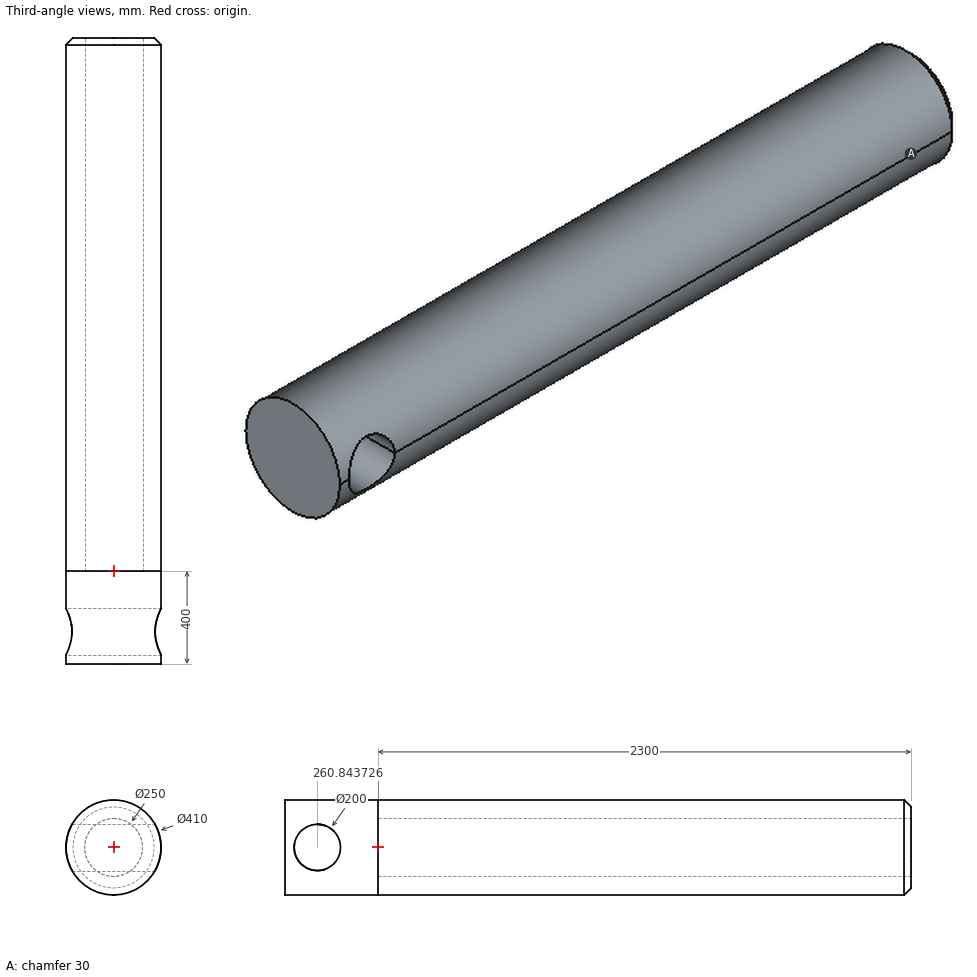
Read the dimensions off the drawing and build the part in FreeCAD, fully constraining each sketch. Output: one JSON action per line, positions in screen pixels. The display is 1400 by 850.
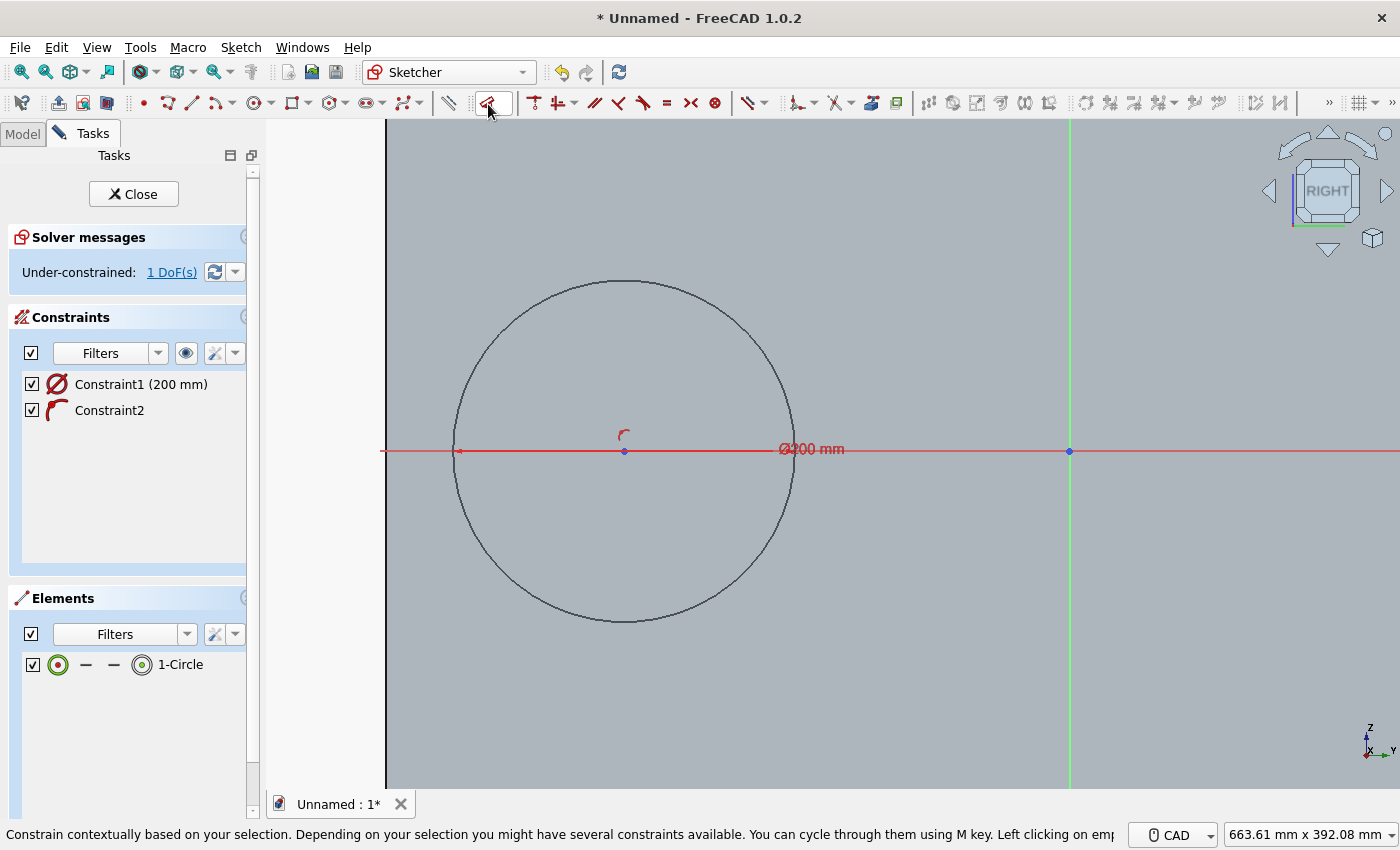
{"action": "left_click", "coordinate": [624, 451]}
{"action": "left_click", "coordinate": [847, 485]}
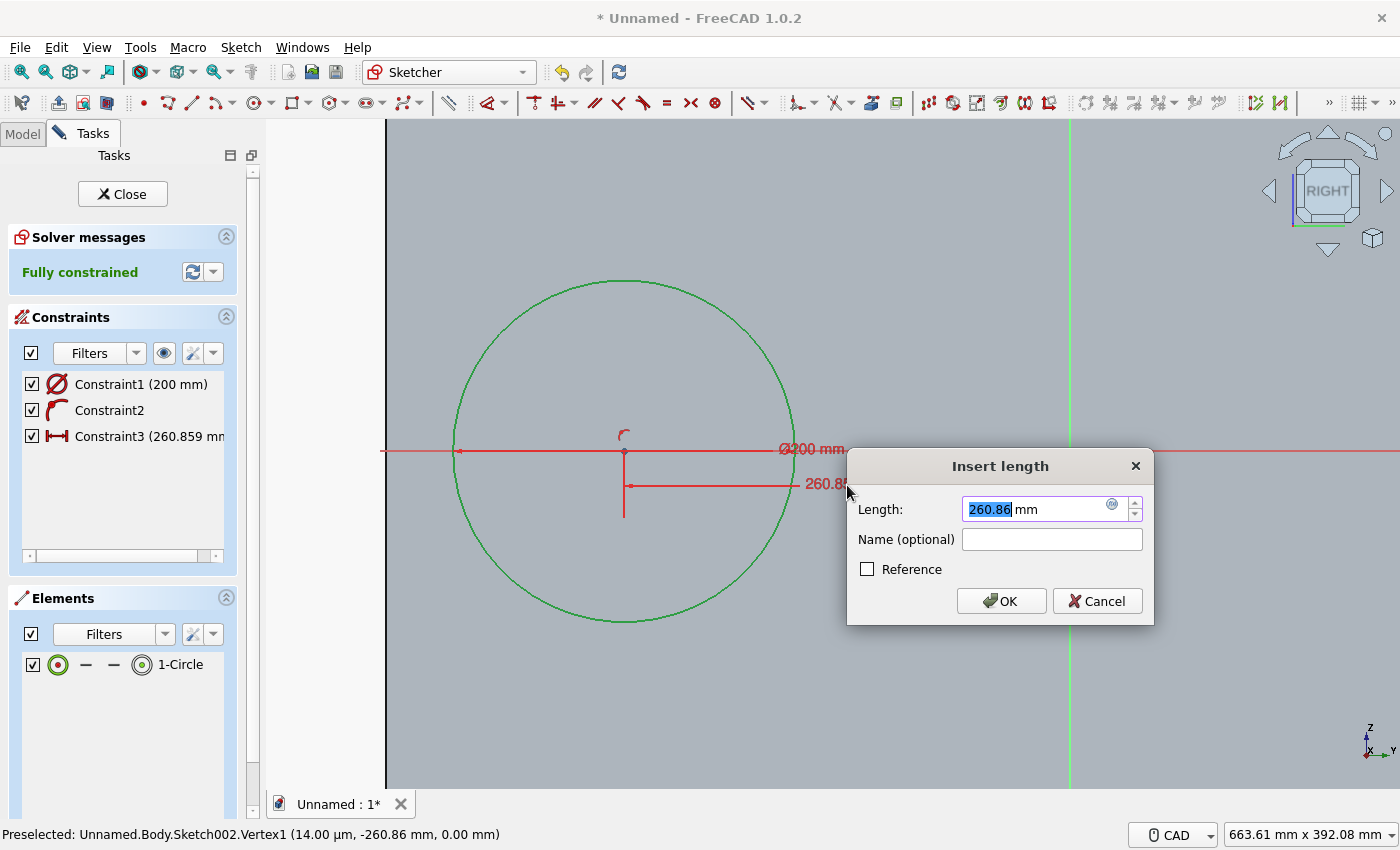
{"action": "type", "text": "260.843726"}
{"action": "key", "text": "Return"}
{"action": "key", "text": "Escape"}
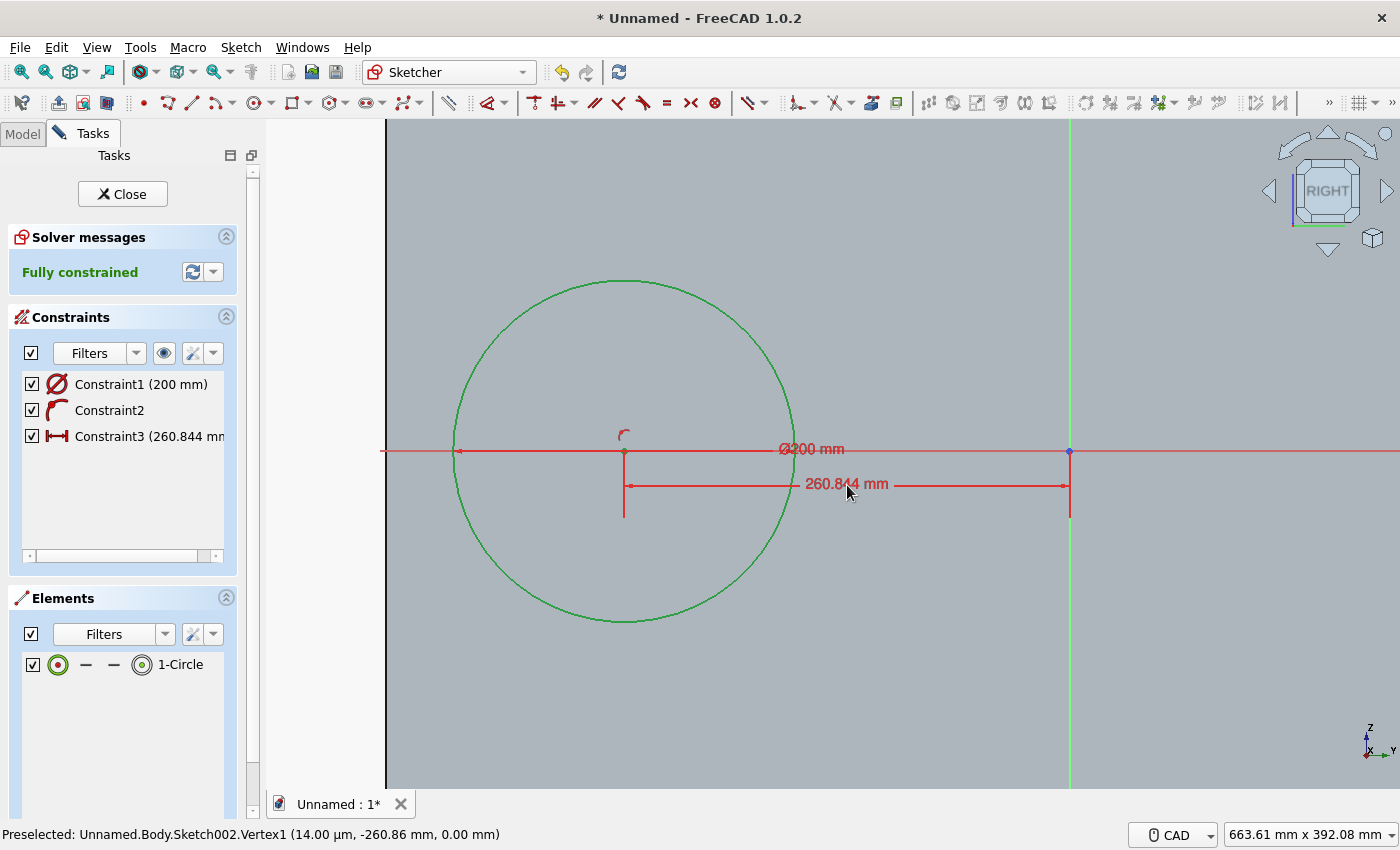
{"action": "left_click", "coordinate": [123, 194]}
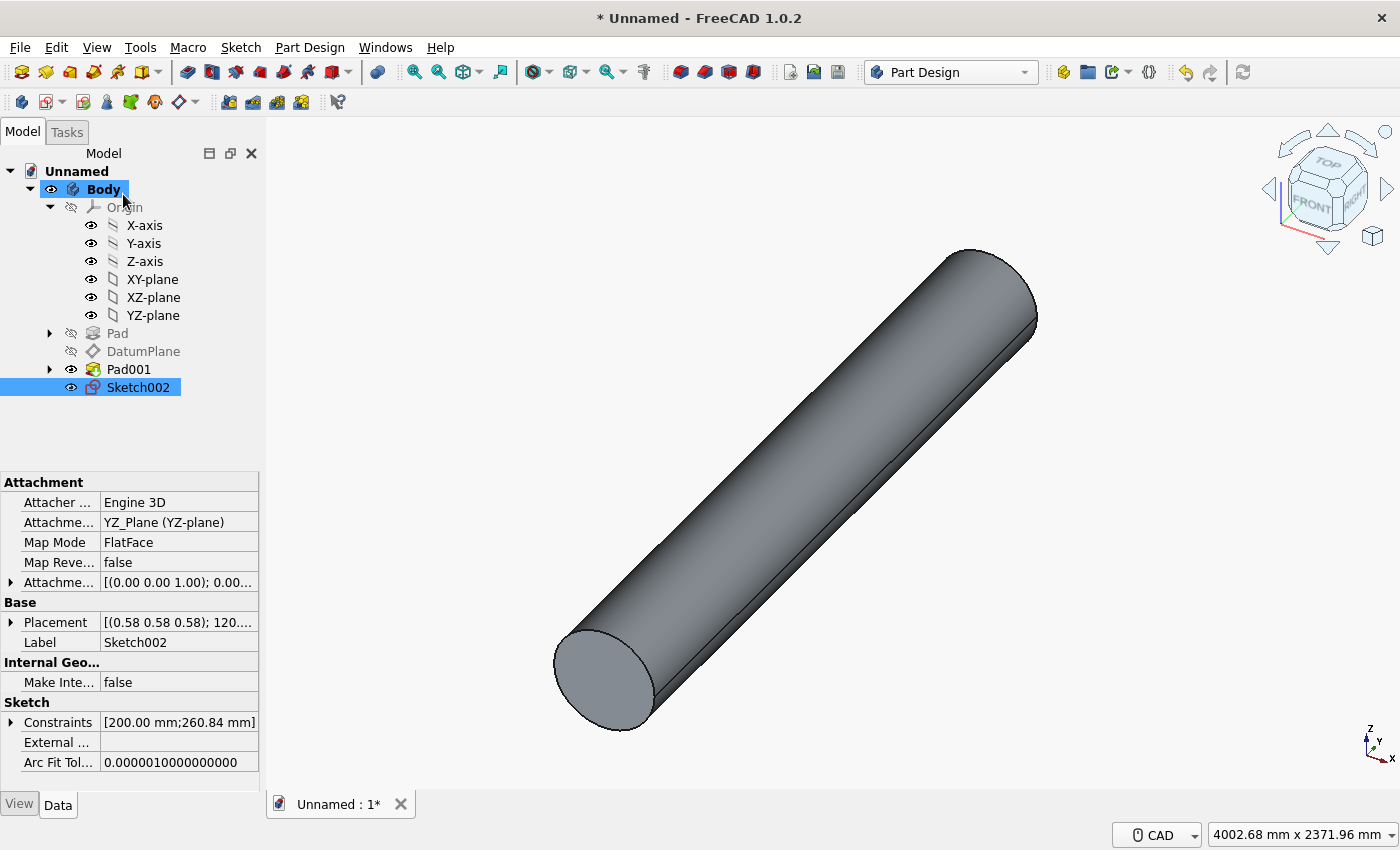
{"action": "left_click", "coordinate": [188, 72]}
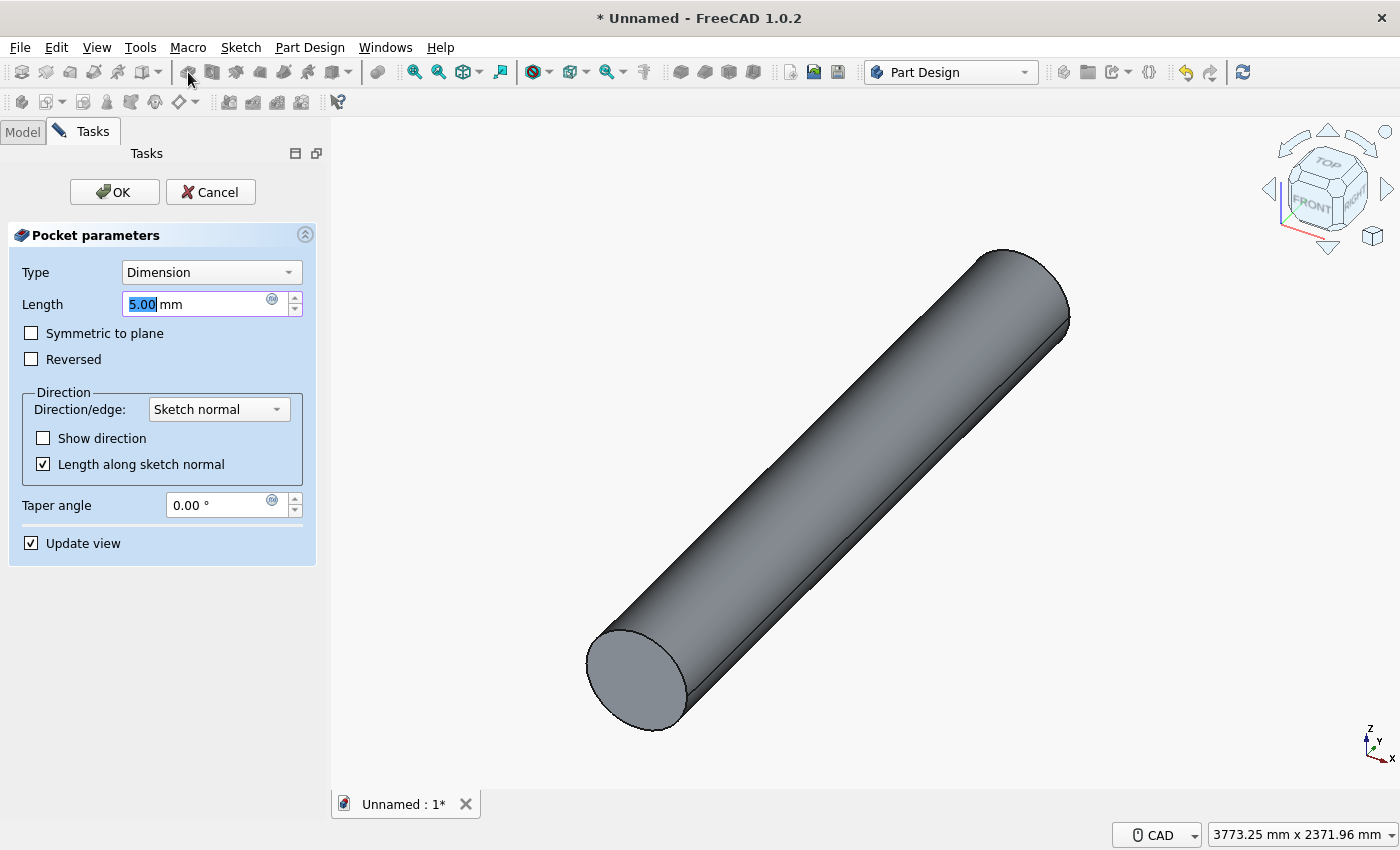
{"action": "left_click", "coordinate": [212, 272]}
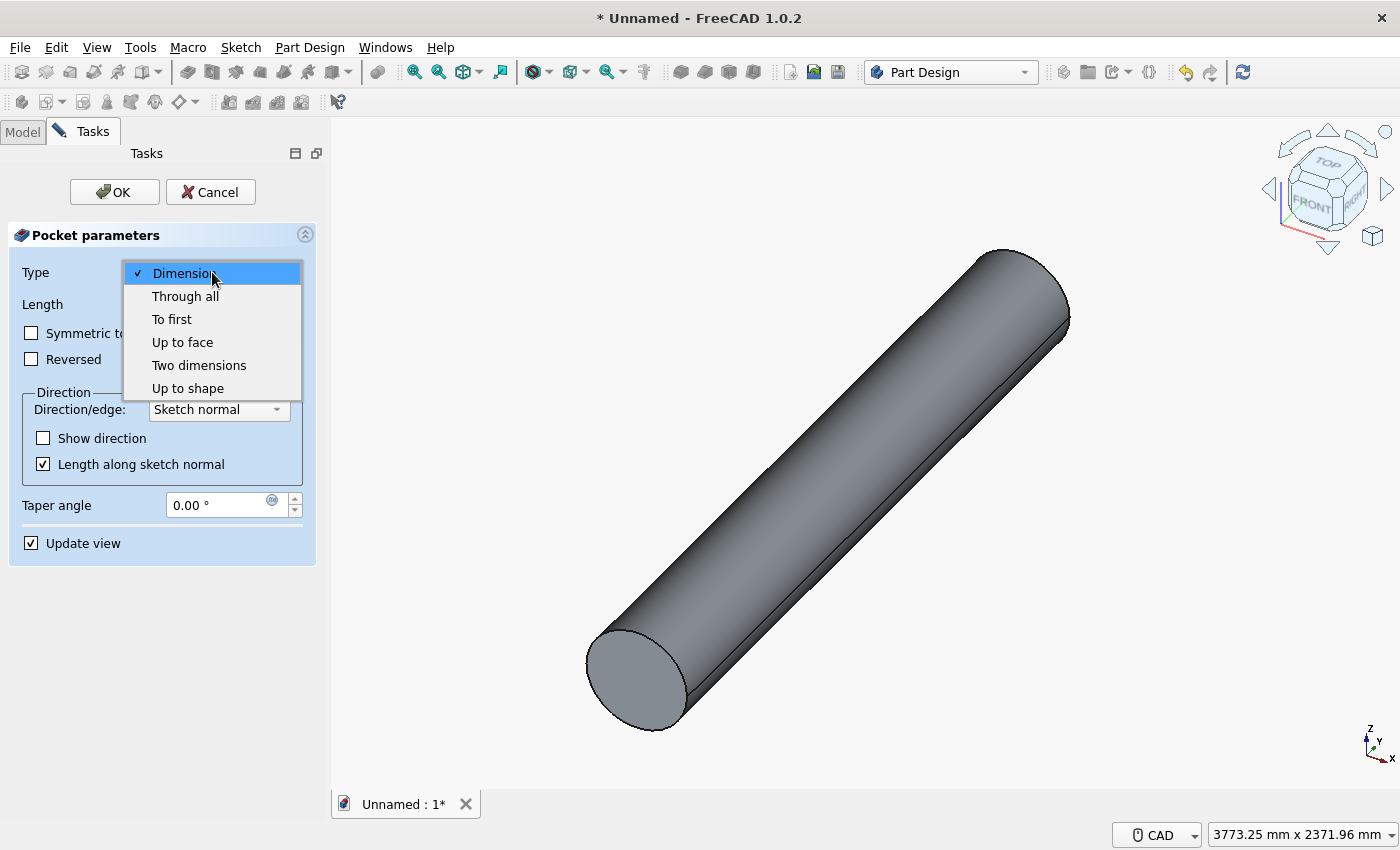
{"action": "left_click", "coordinate": [212, 366]}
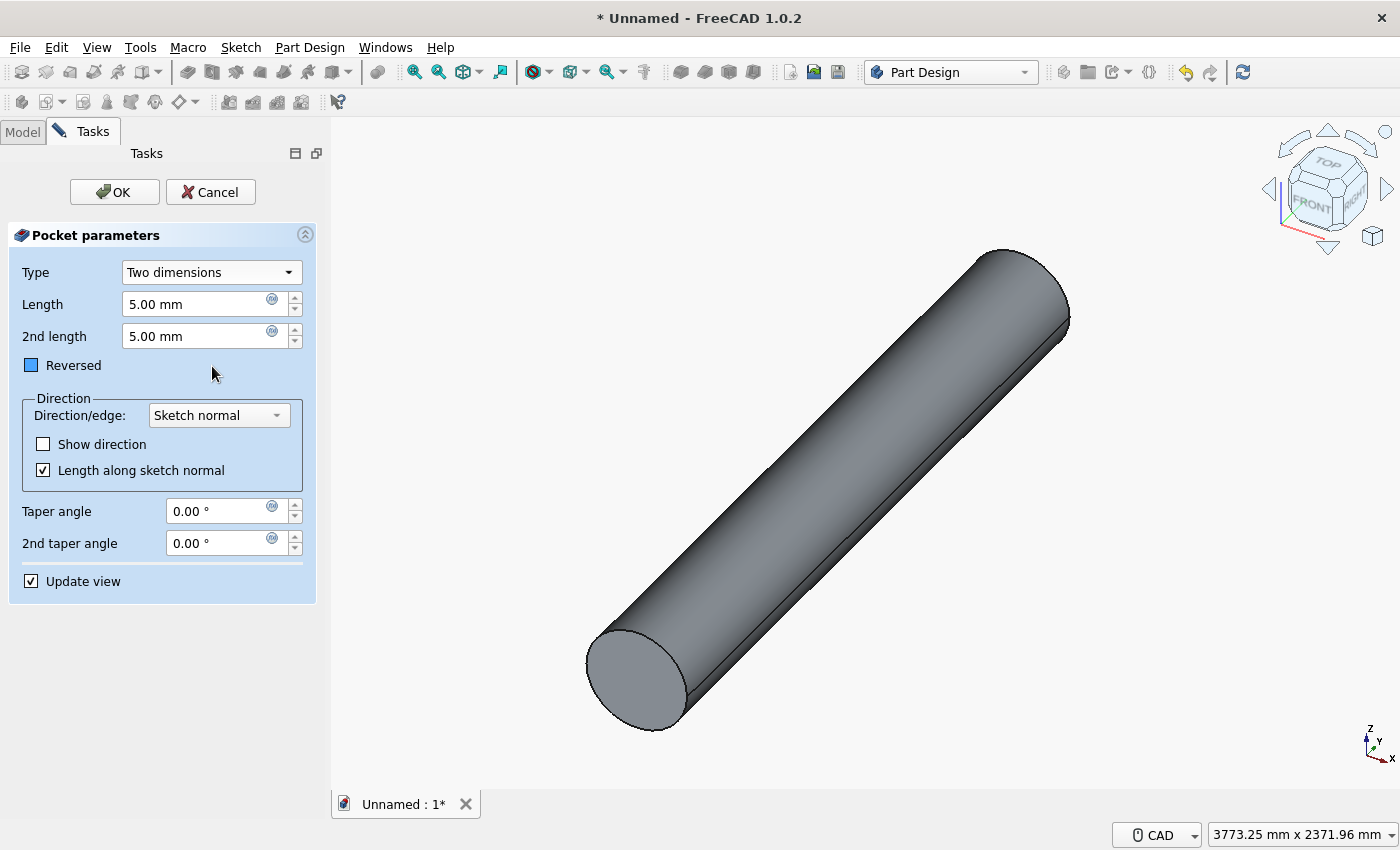
{"action": "triple_click", "coordinate": [204, 304]}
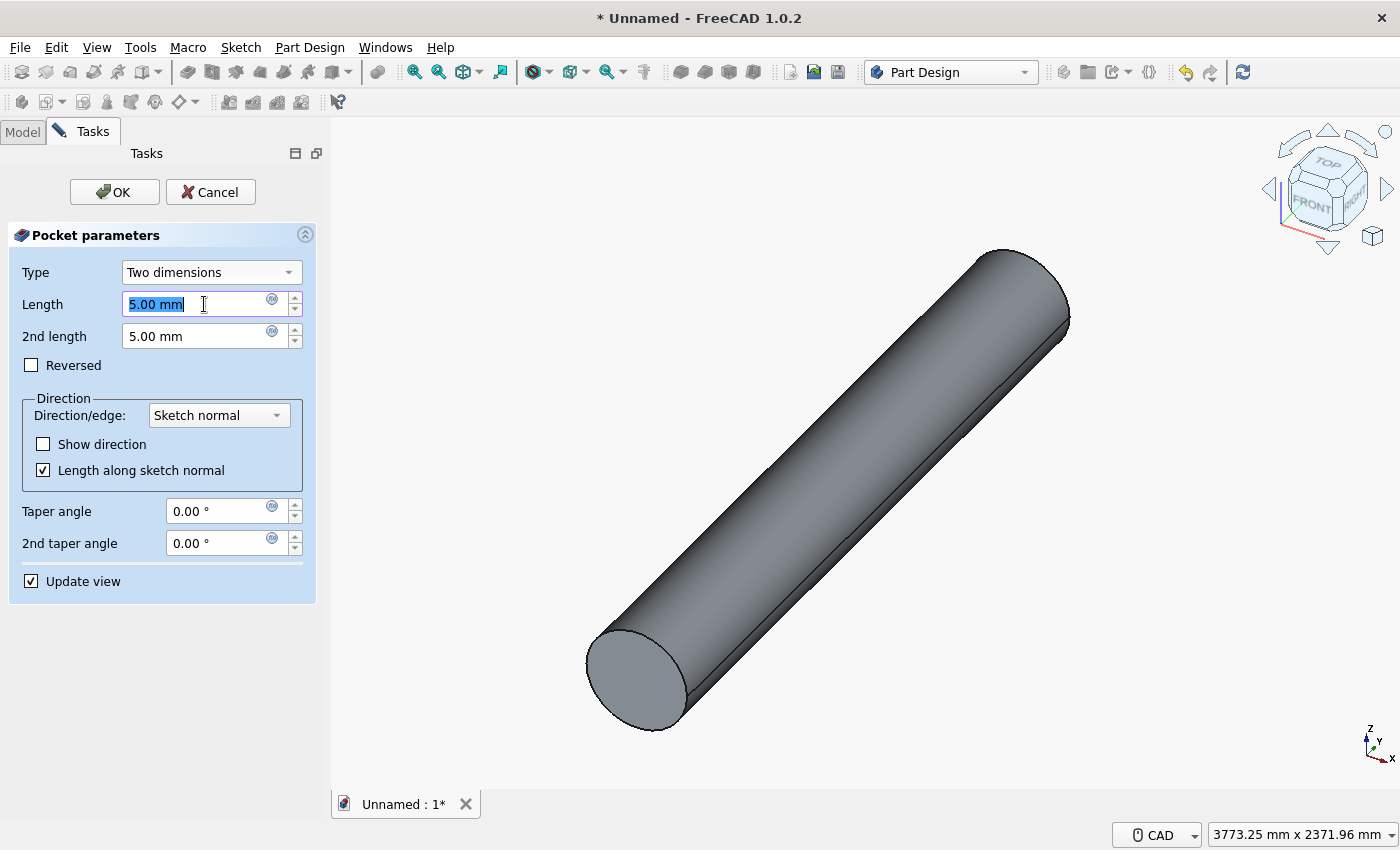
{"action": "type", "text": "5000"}
{"action": "key", "text": "Tab"}